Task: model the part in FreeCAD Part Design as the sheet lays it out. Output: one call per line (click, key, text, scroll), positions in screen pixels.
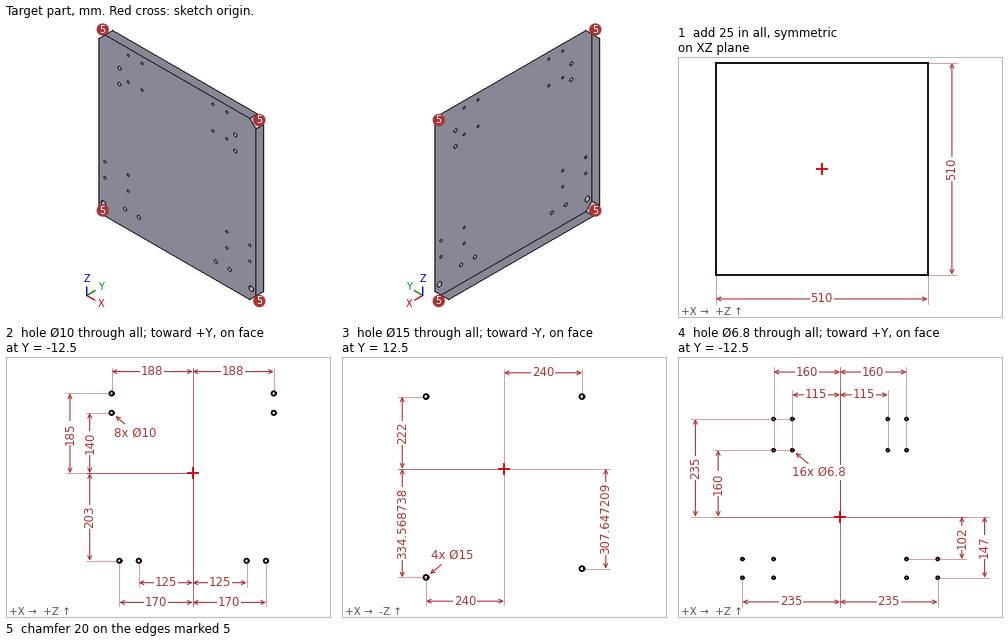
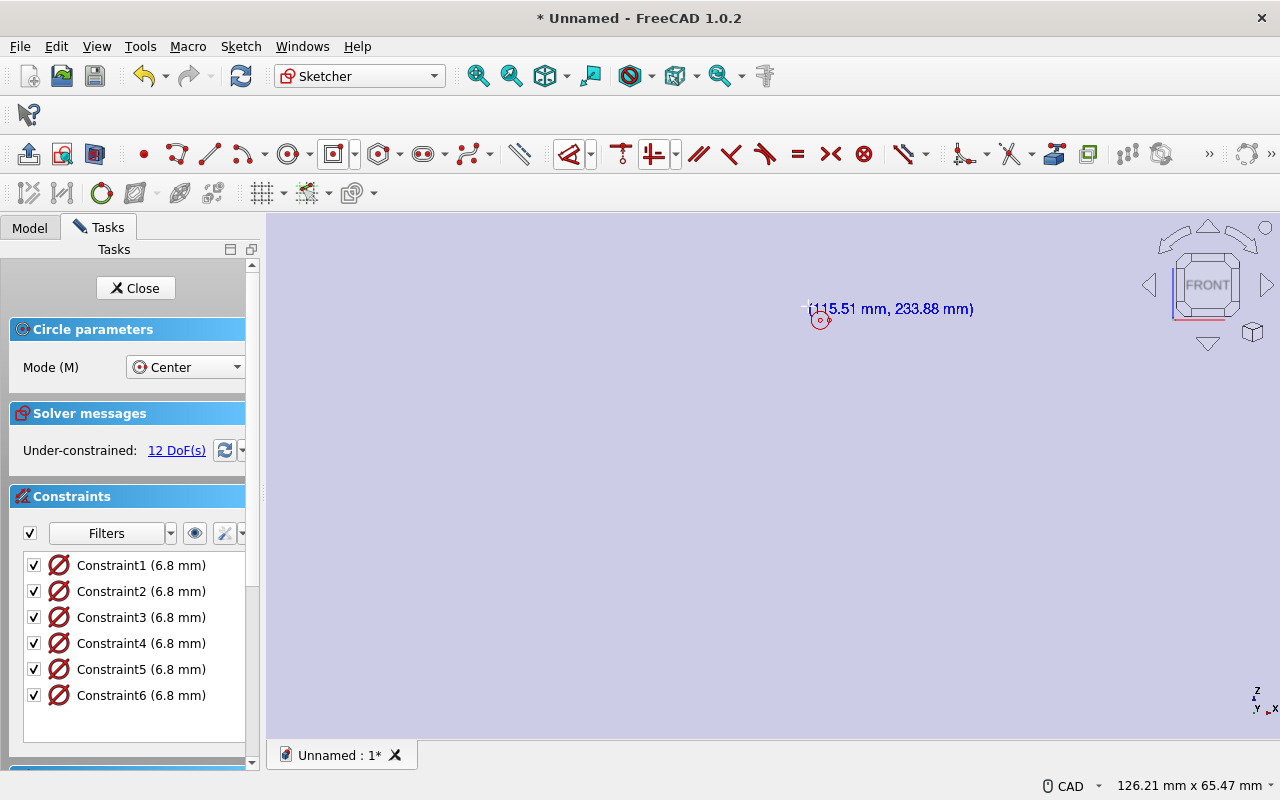
scroll(808, 306, down, 11)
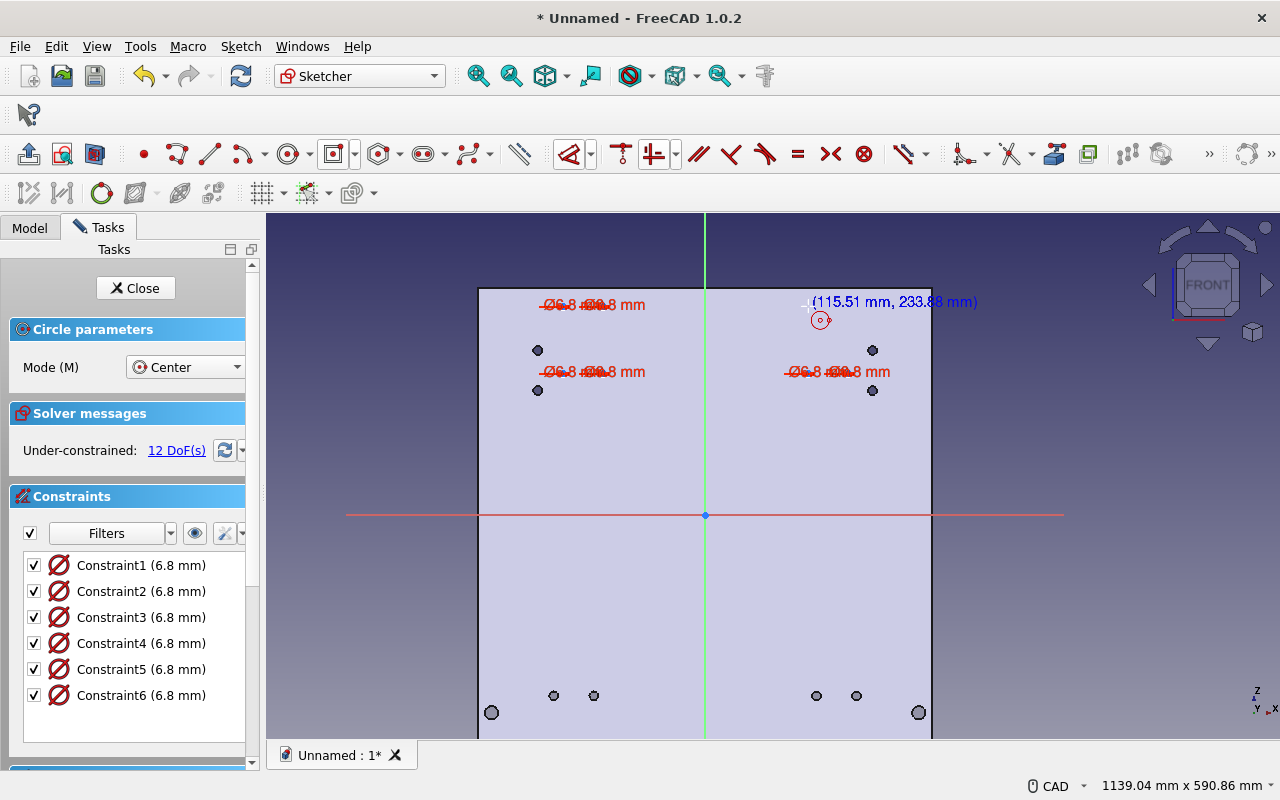
click(808, 306)
move(810, 304)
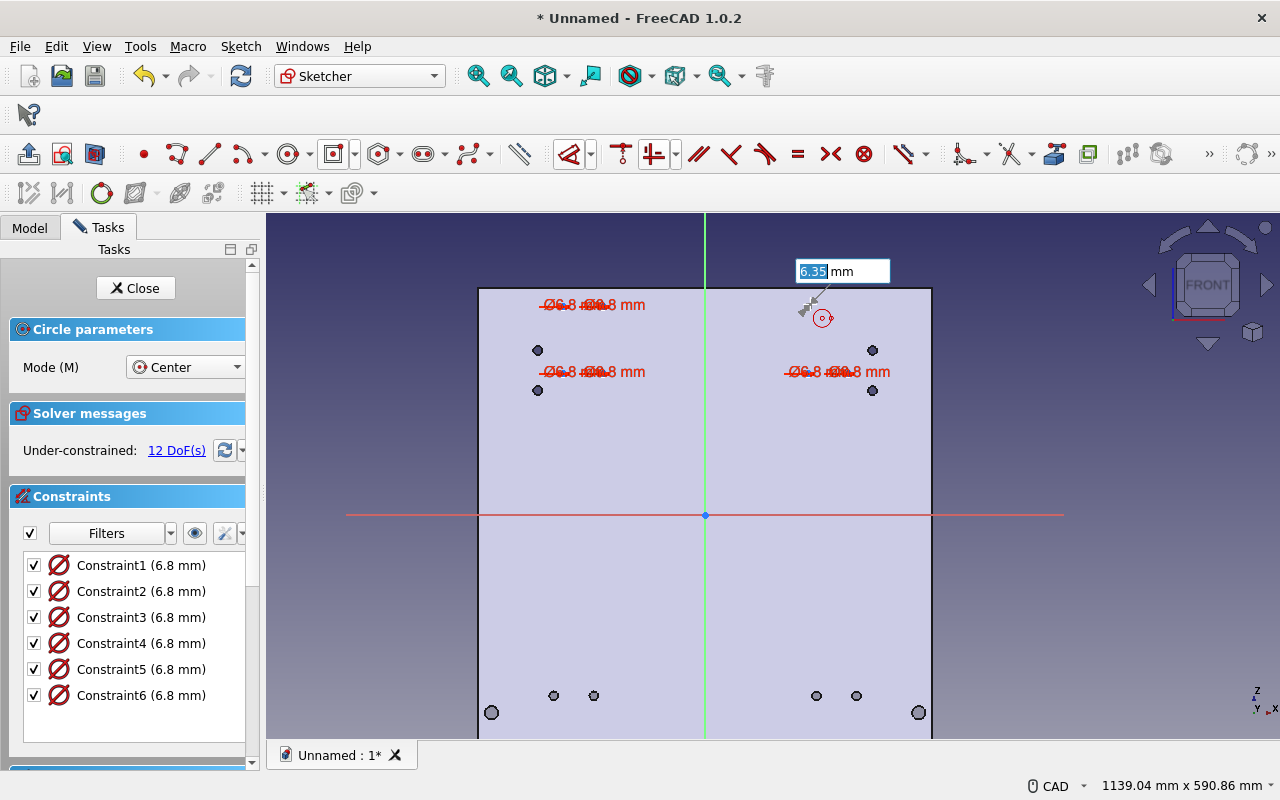
text(6.8)
key(Return)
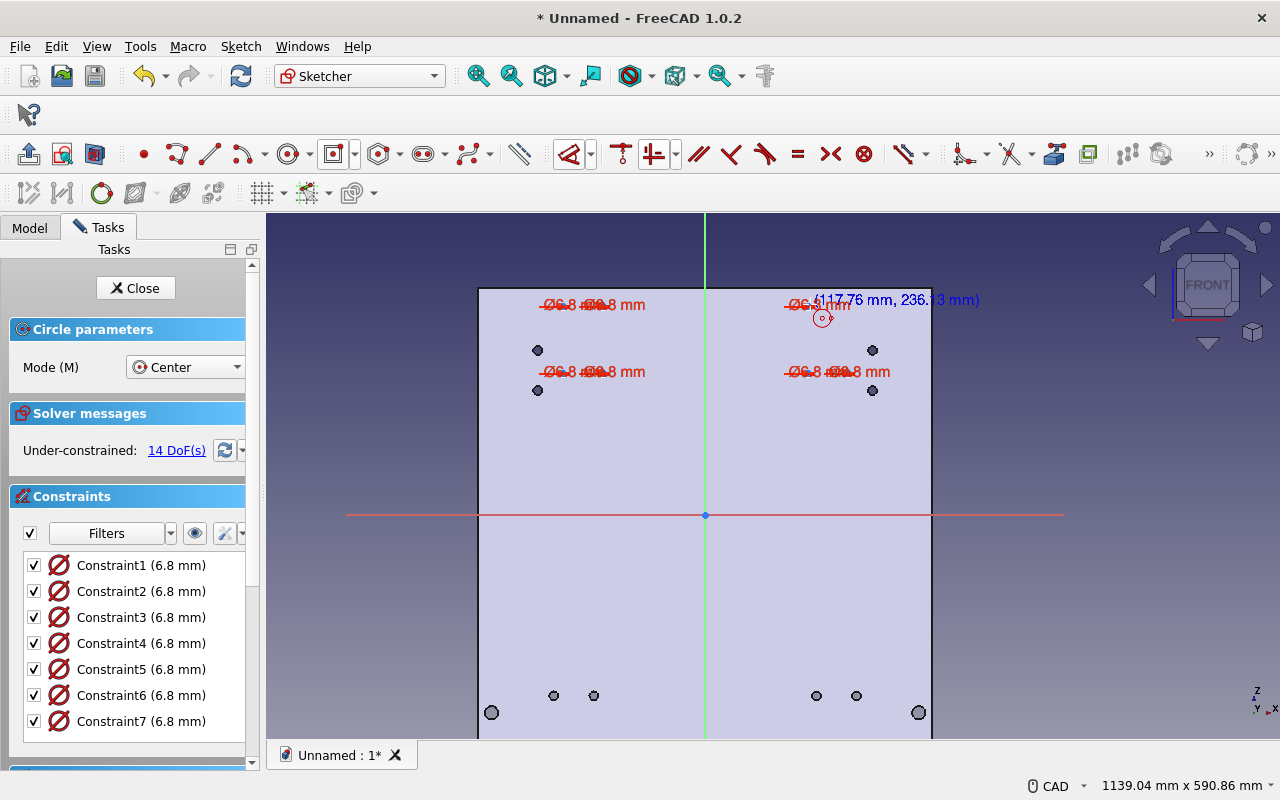
scroll(848, 306, up, 11)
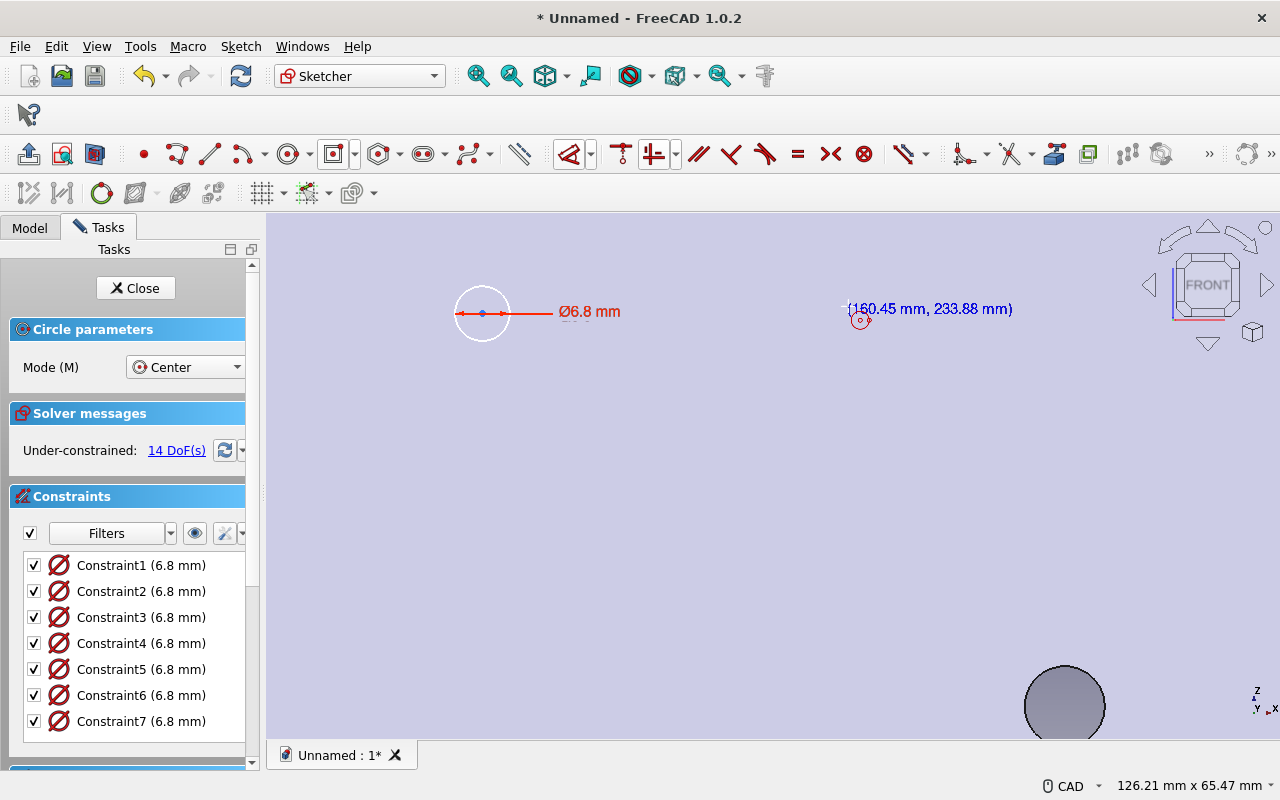
scroll(848, 306, down, 11)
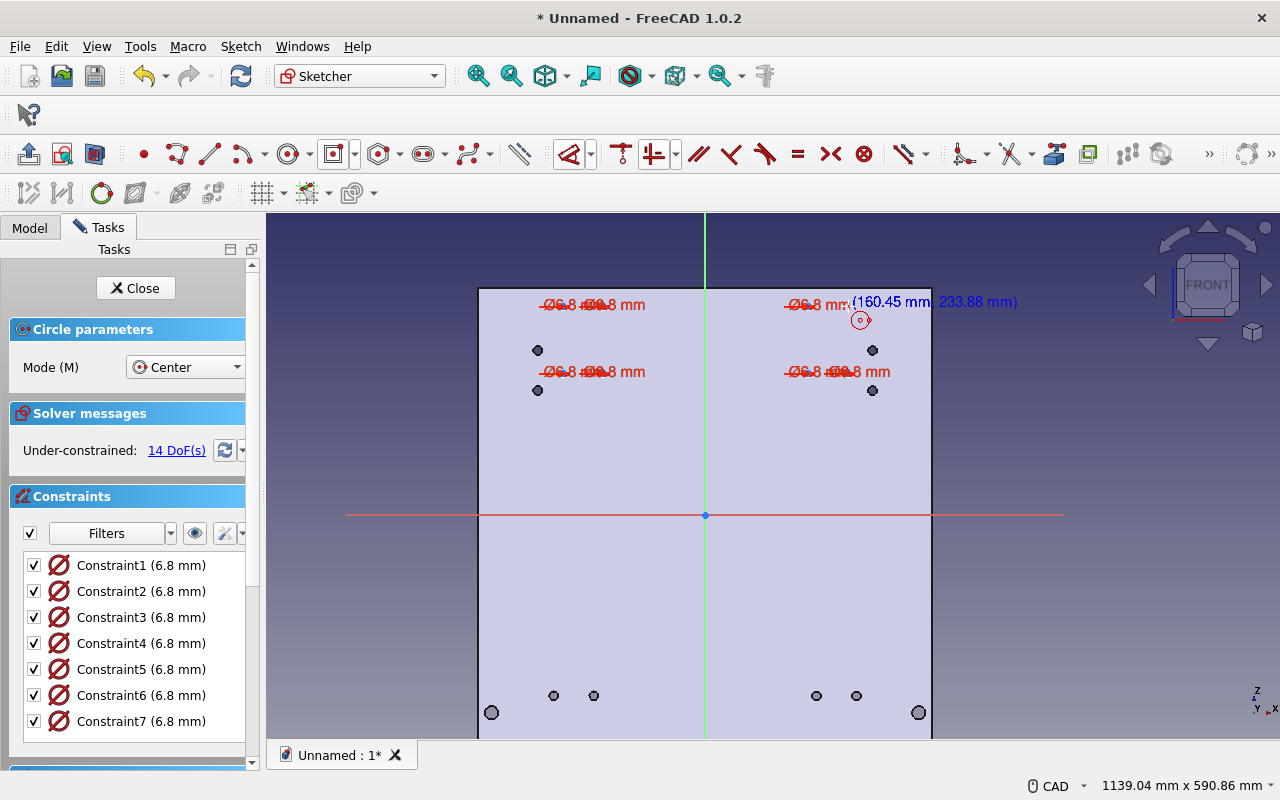
click(848, 306)
move(850, 304)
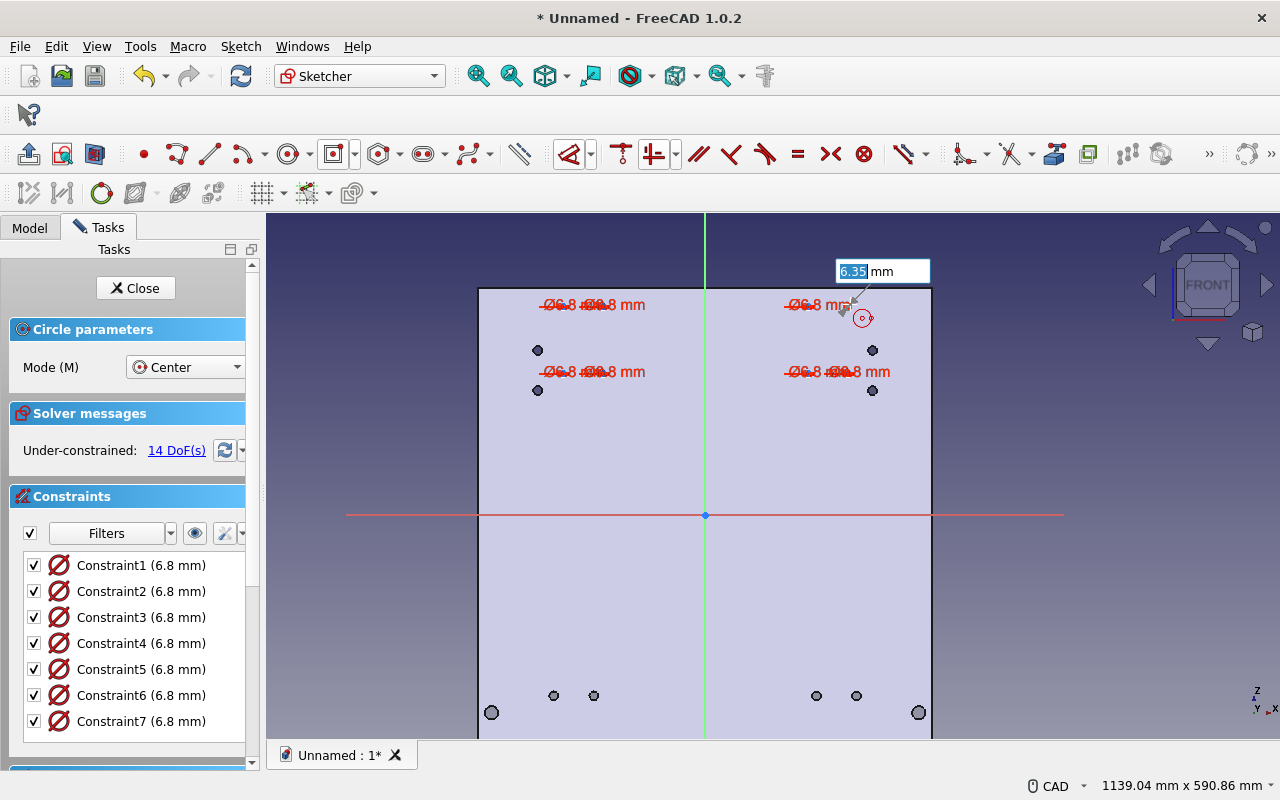
text(6.8)
key(Return)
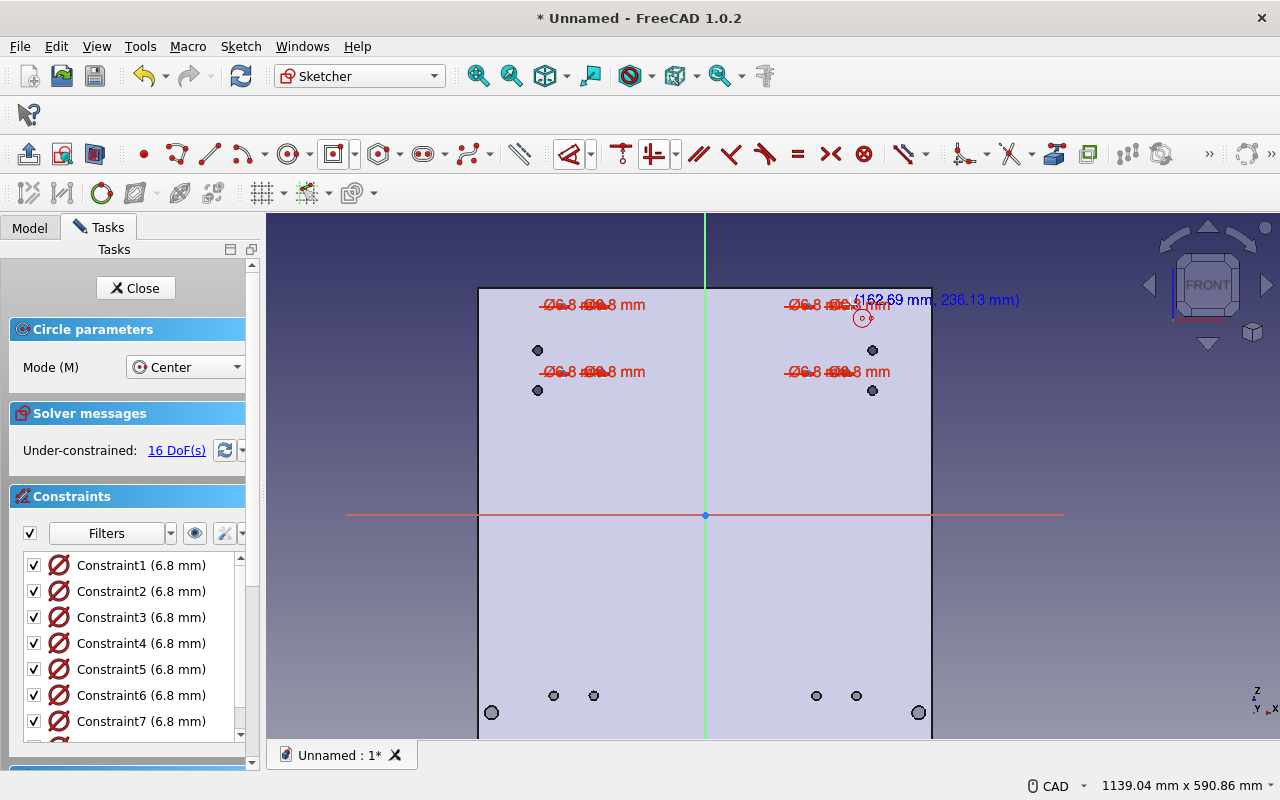
scroll(914, 646, up, 11)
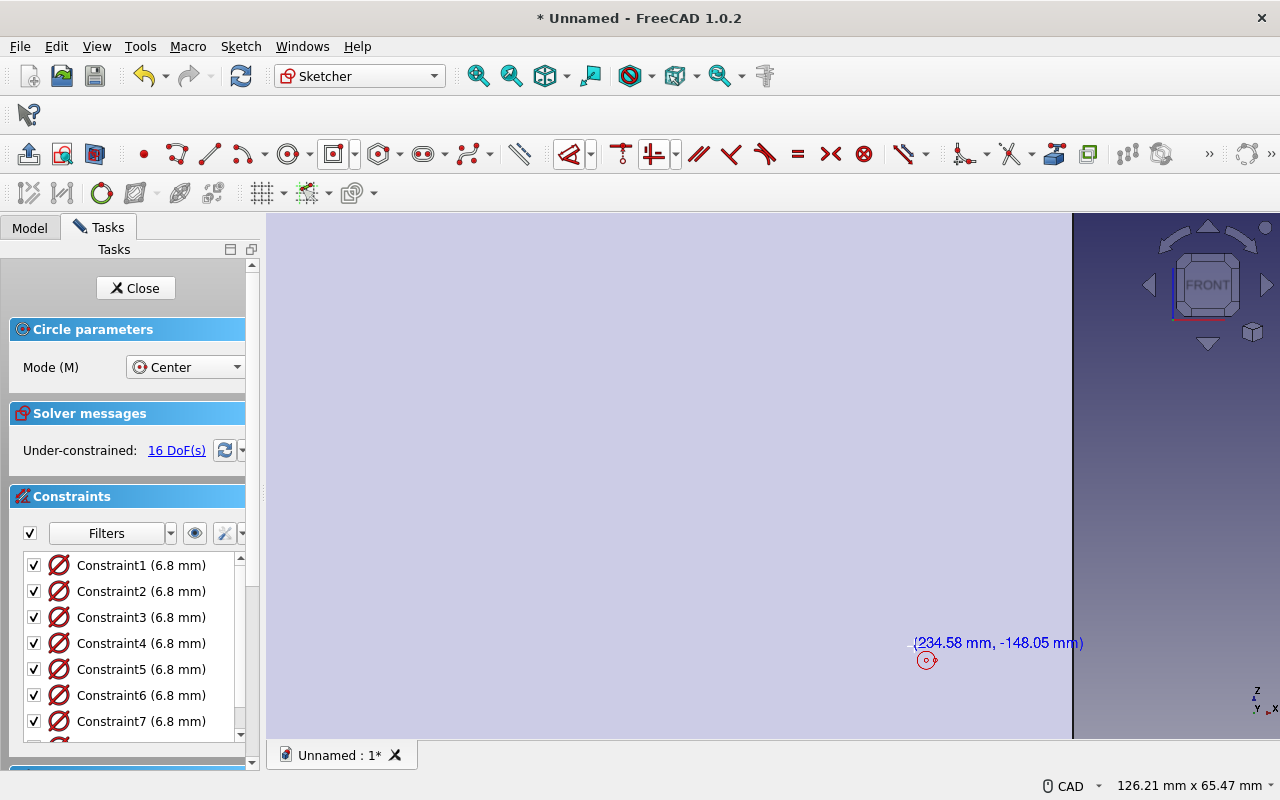
scroll(914, 647, down, 11)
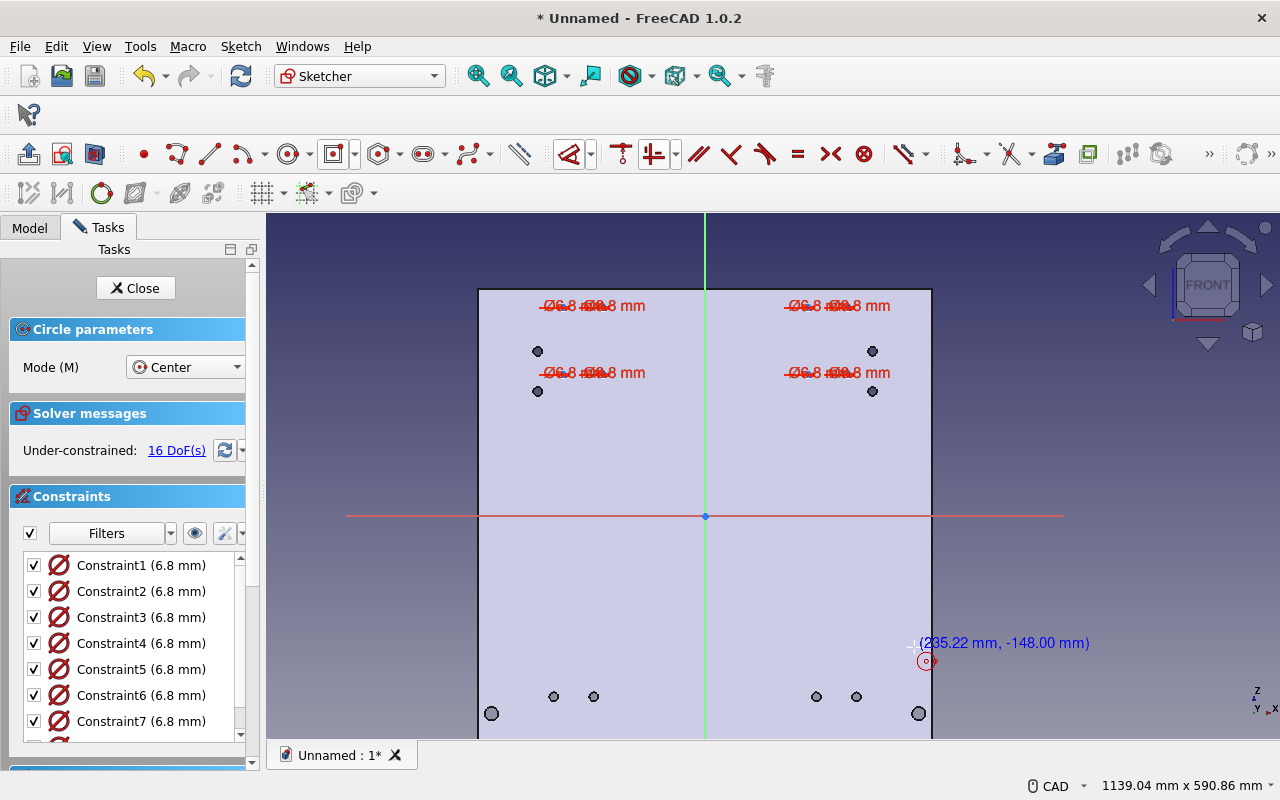
click(914, 647)
move(917, 645)